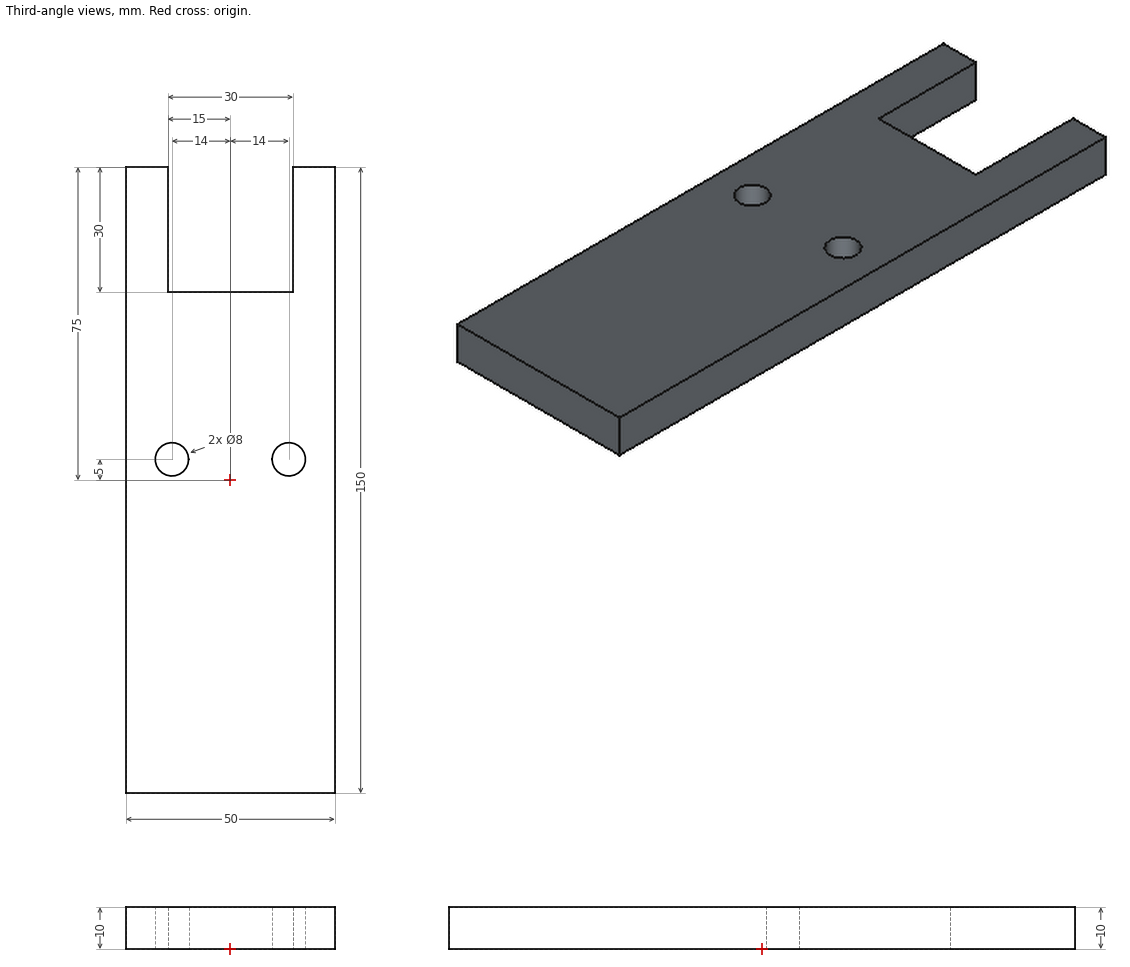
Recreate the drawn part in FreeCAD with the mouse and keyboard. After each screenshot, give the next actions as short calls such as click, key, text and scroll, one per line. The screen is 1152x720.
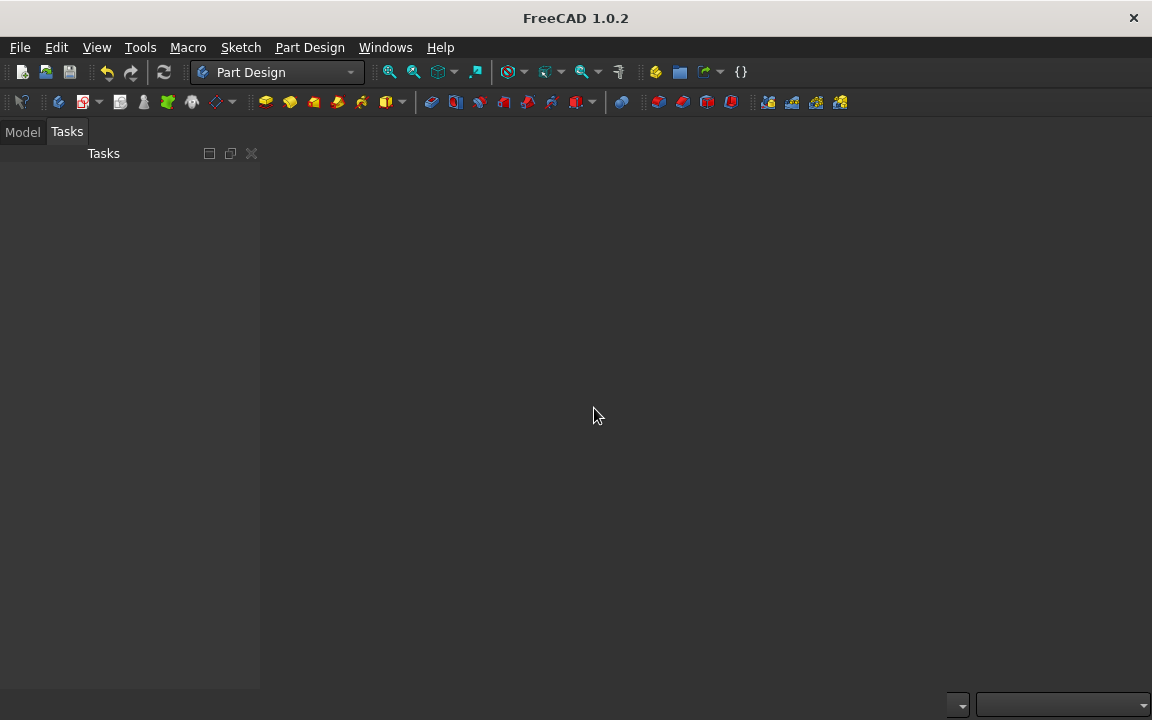
key(ctrl+n)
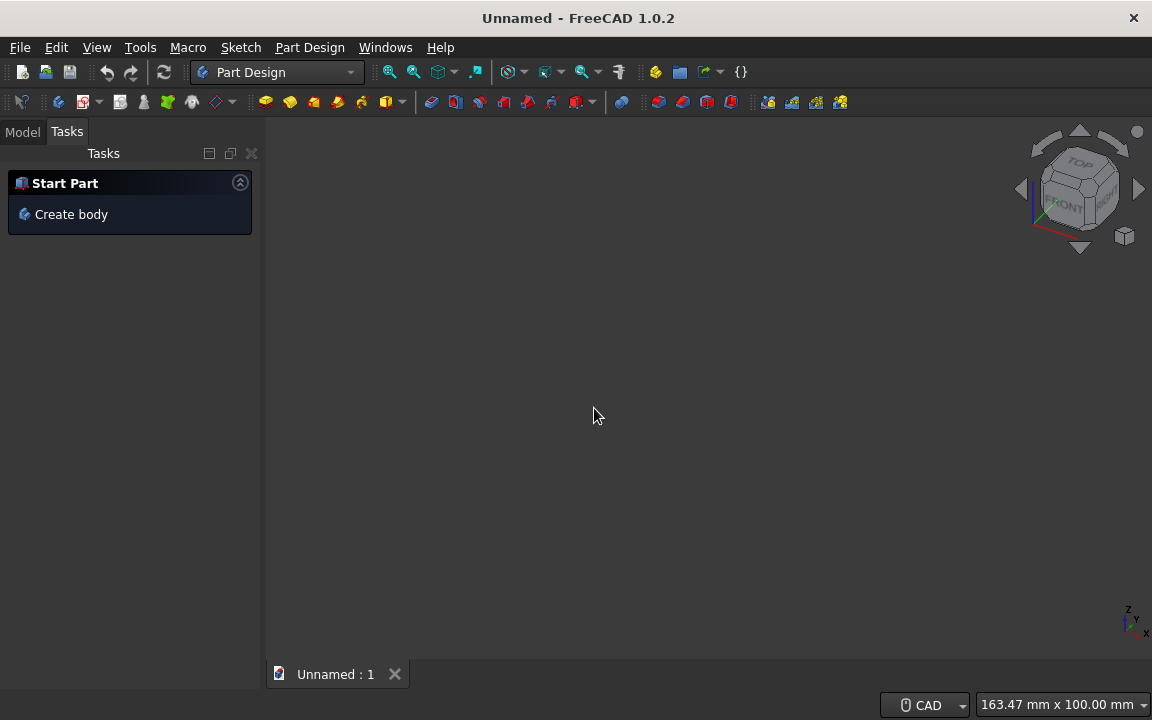
click(84, 102)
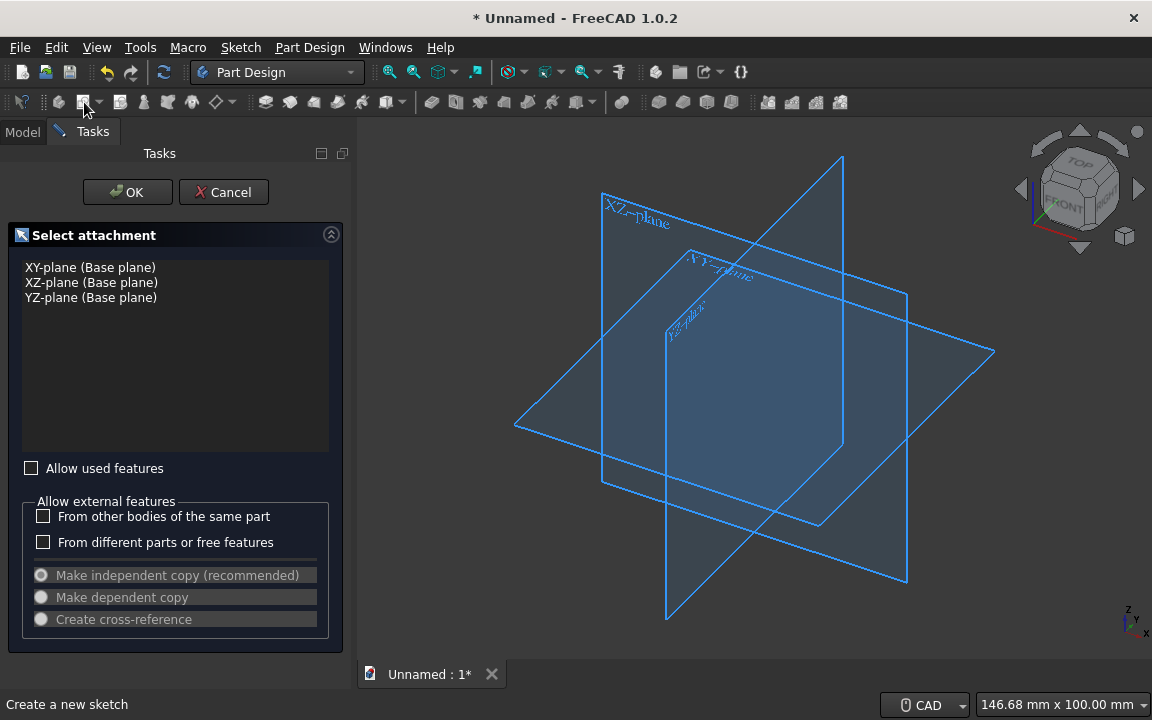
click(82, 268)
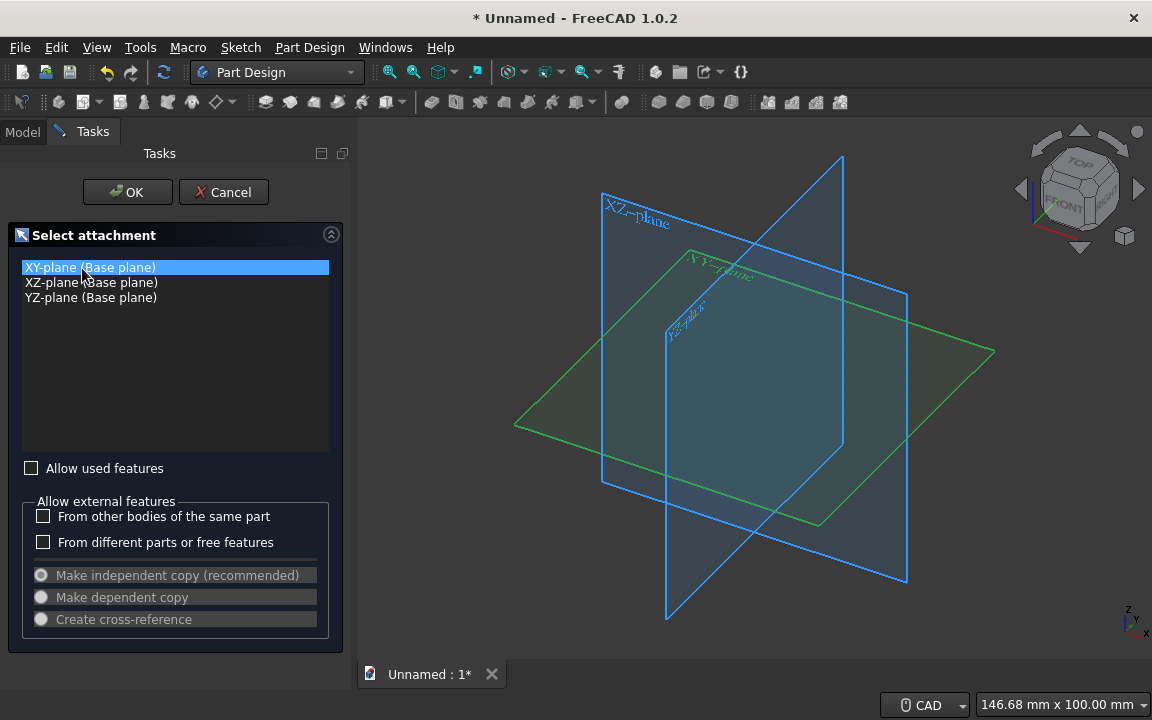
click(128, 192)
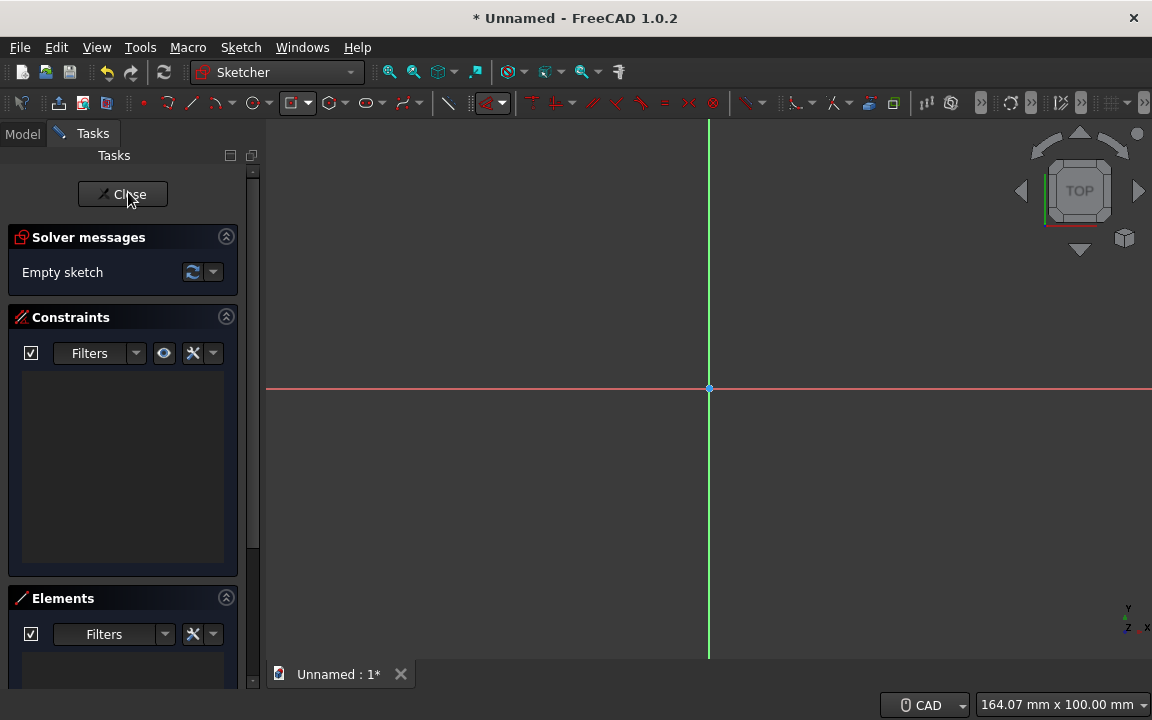
scroll(585, 389, down, 4)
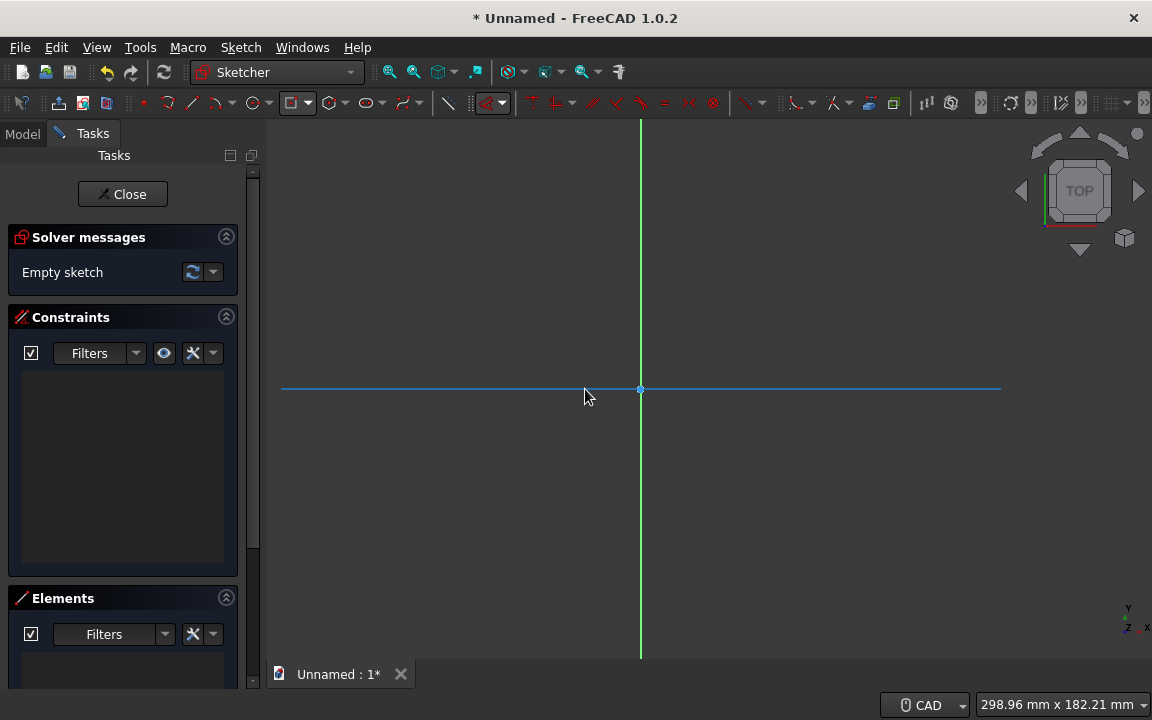
key(g)
key(v)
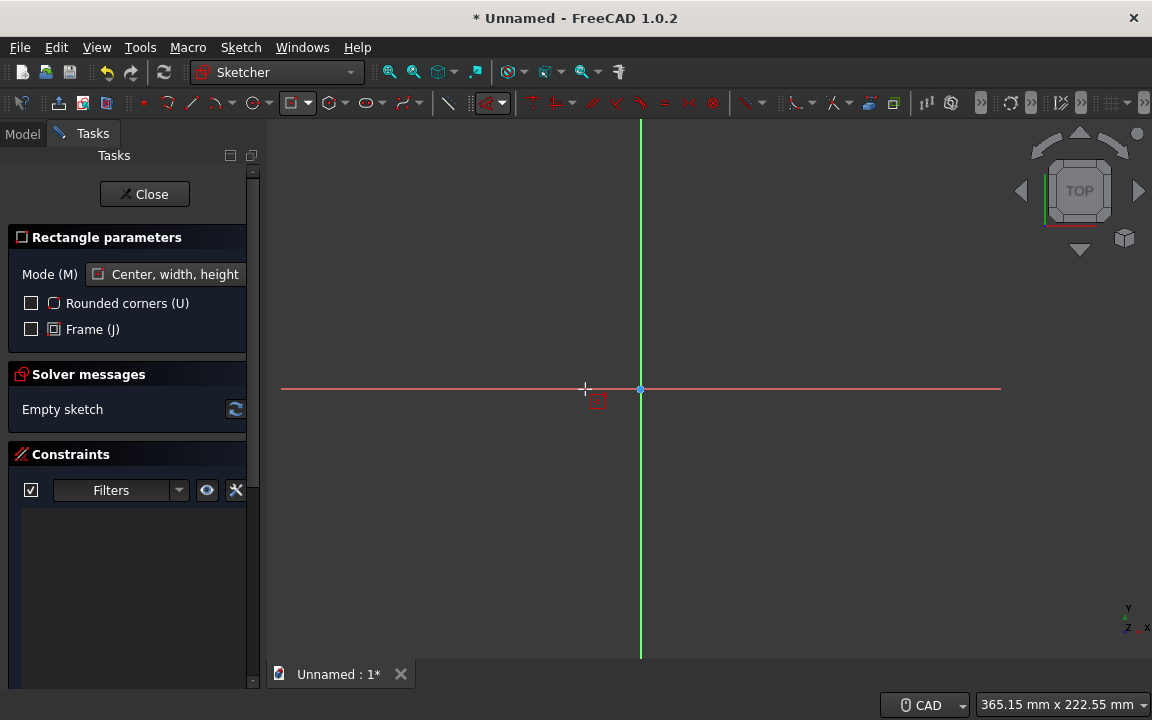
click(641, 389)
click(702, 207)
key(Escape)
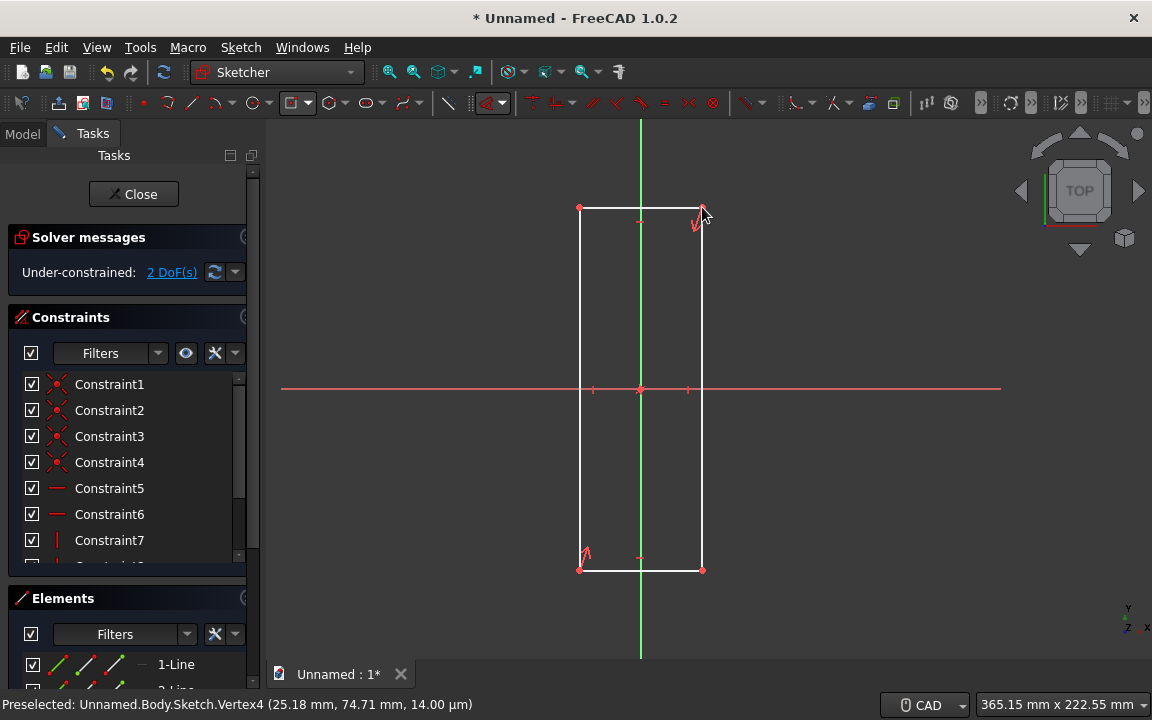
click(486, 104)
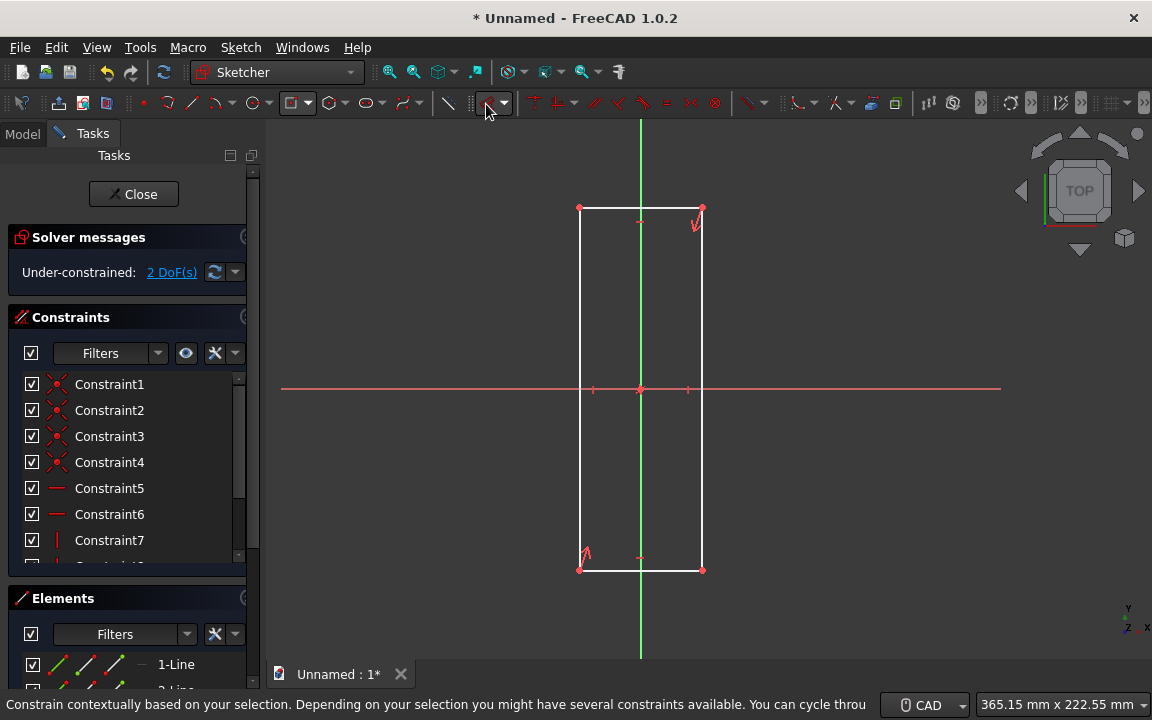
click(616, 571)
click(613, 605)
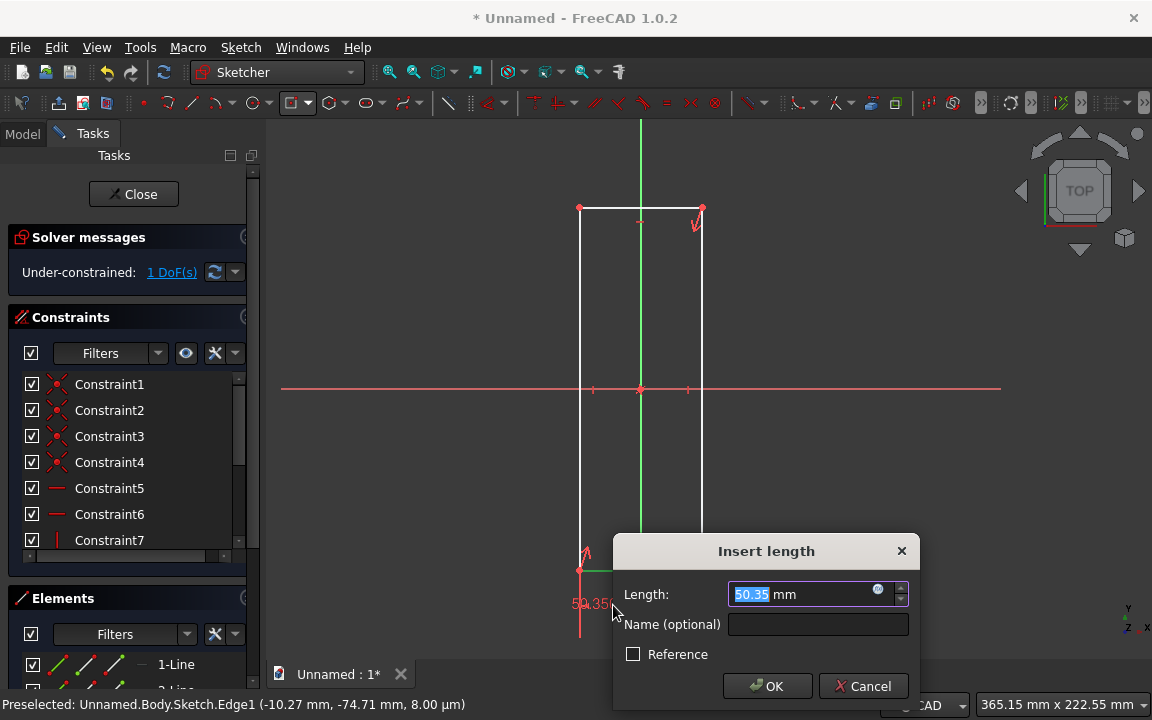
text(50)
key(Return)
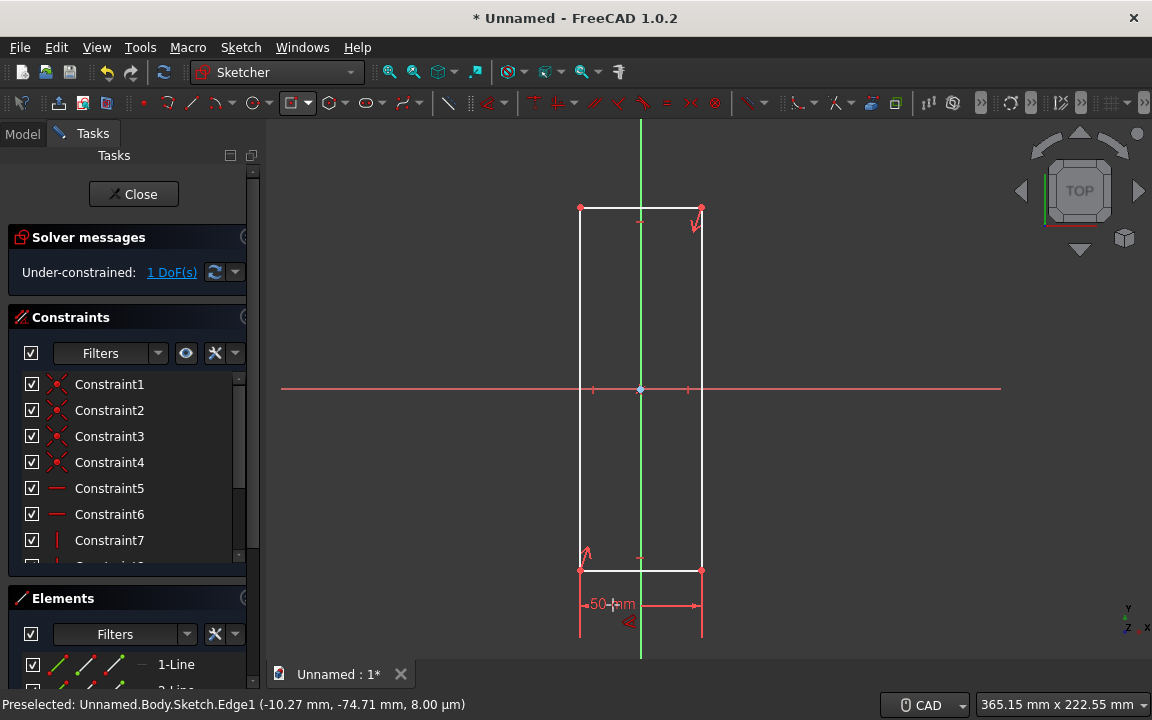
click(702, 462)
click(736, 306)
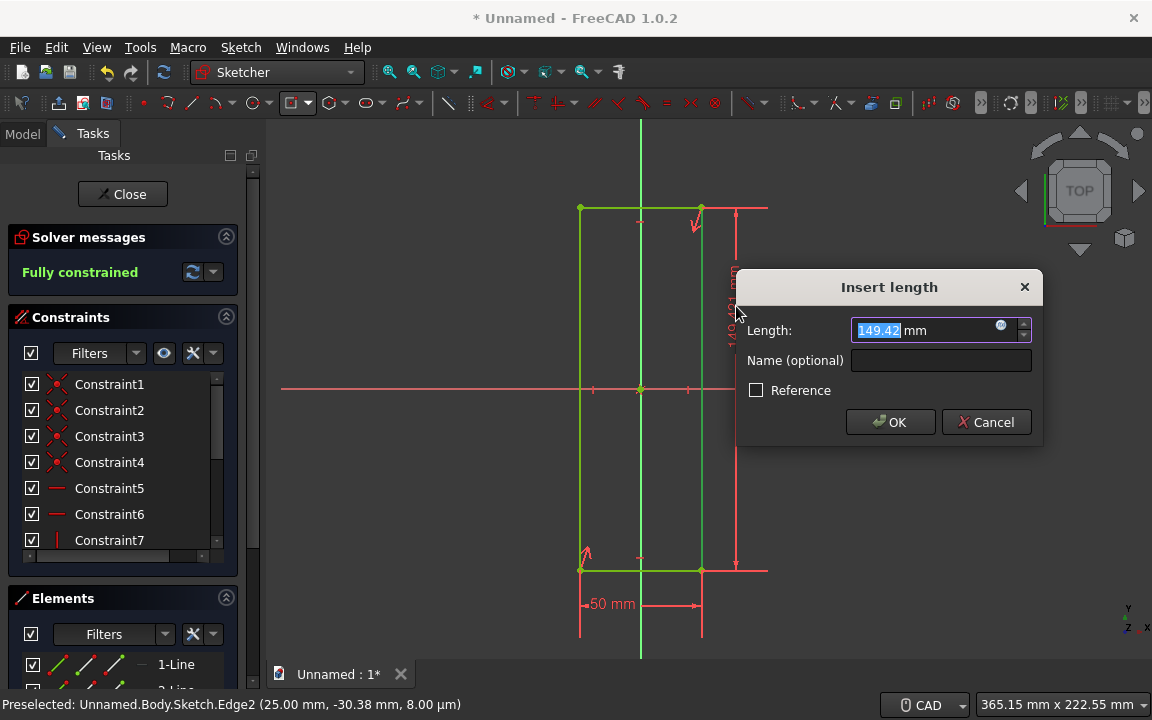
text(150)
key(Return)
key(Escape)